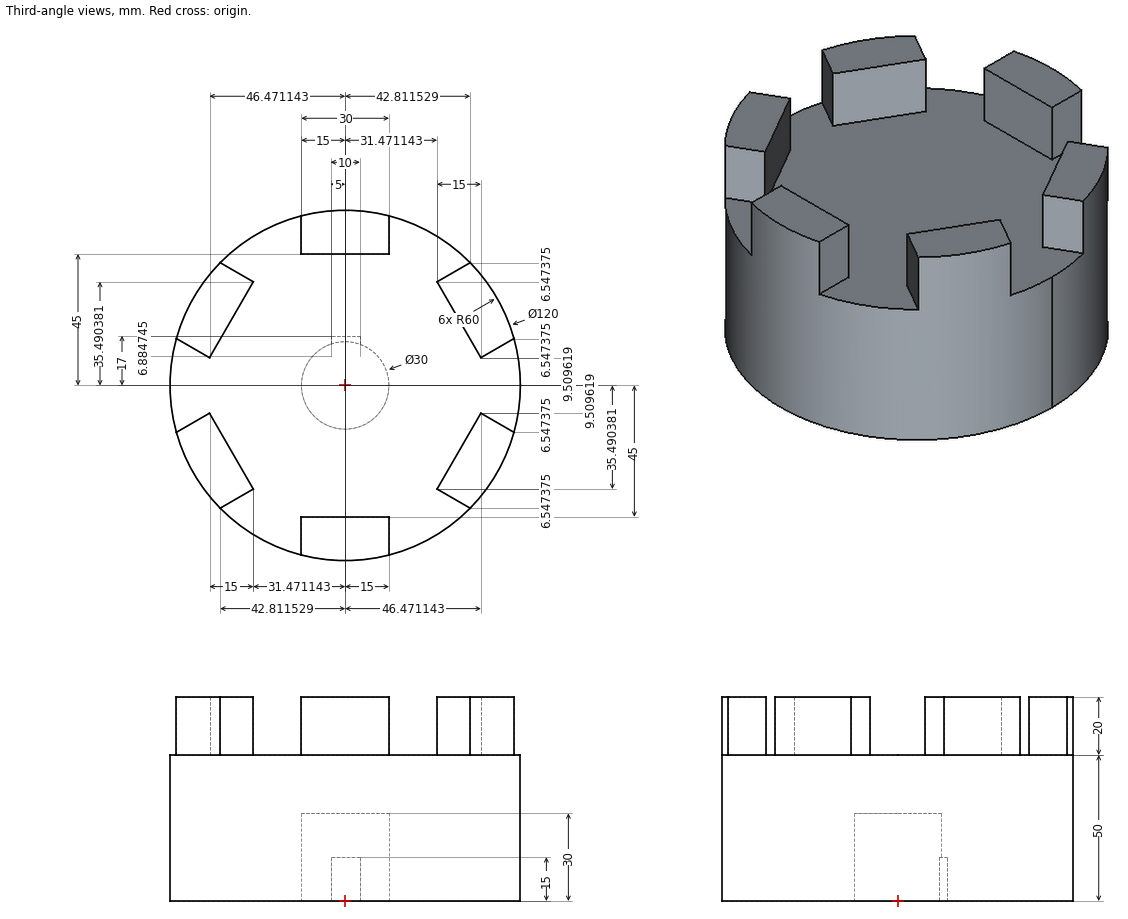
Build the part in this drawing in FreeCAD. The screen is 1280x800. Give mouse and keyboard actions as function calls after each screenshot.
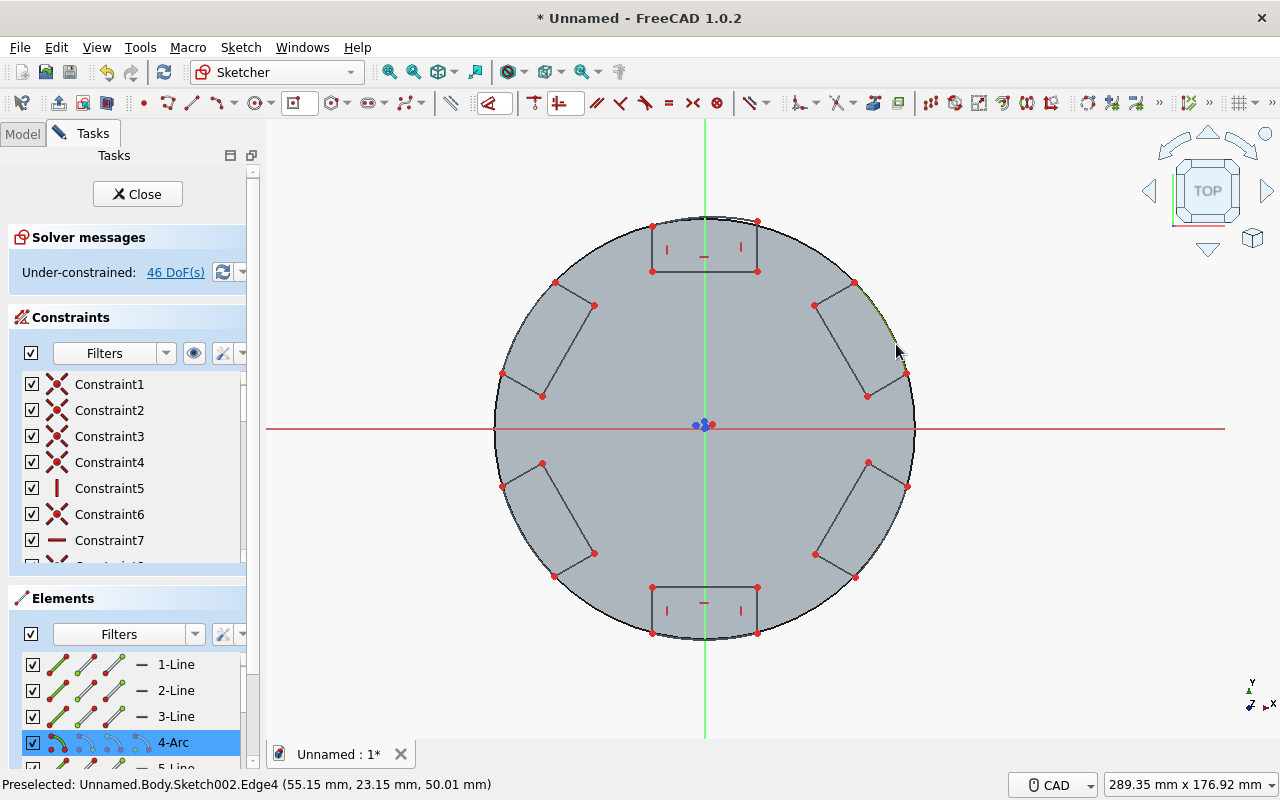
click(875, 552)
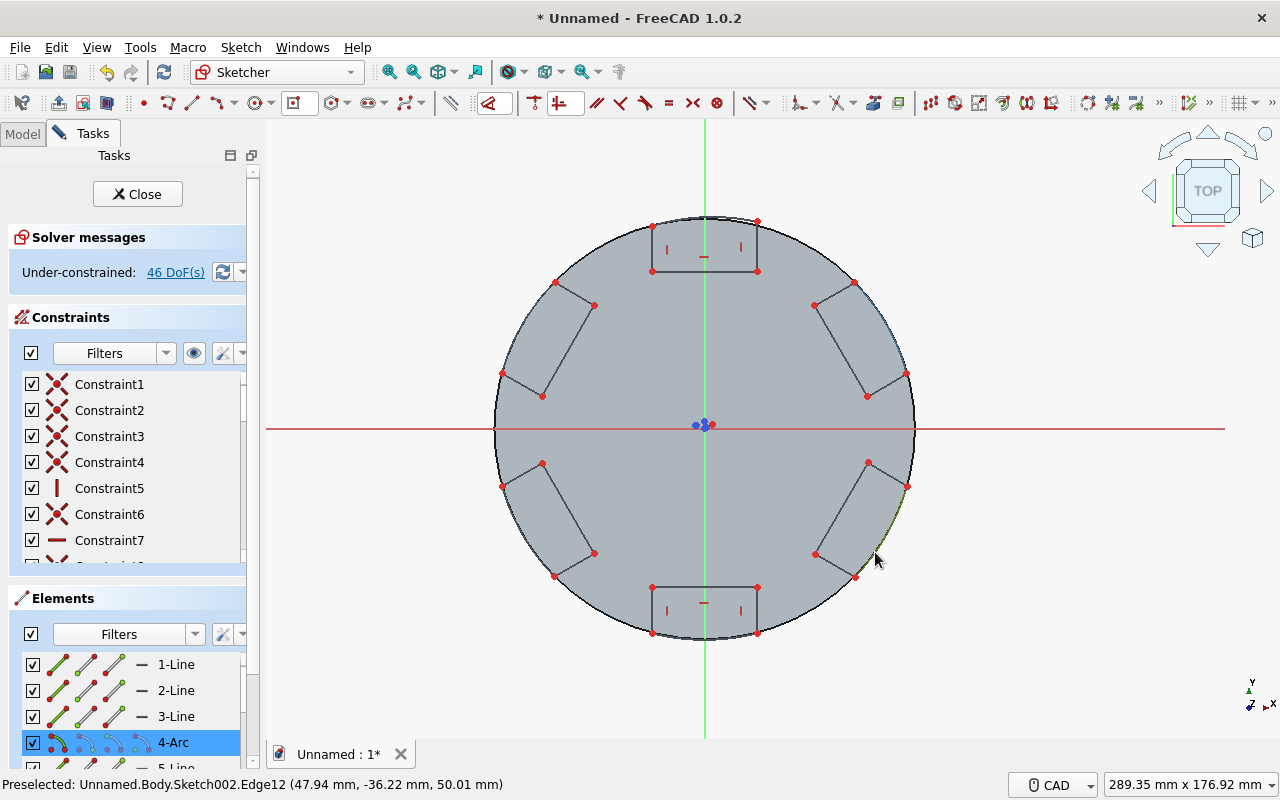
key(c)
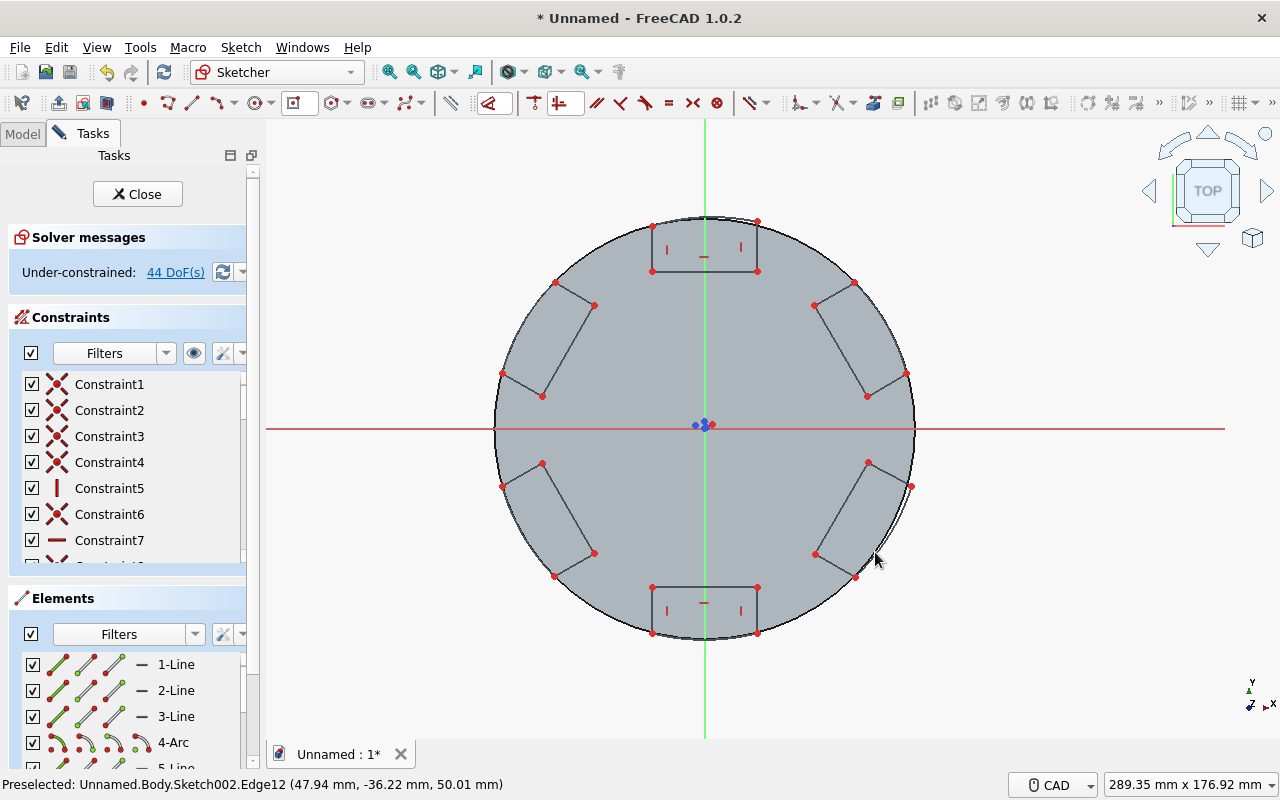
click(896, 344)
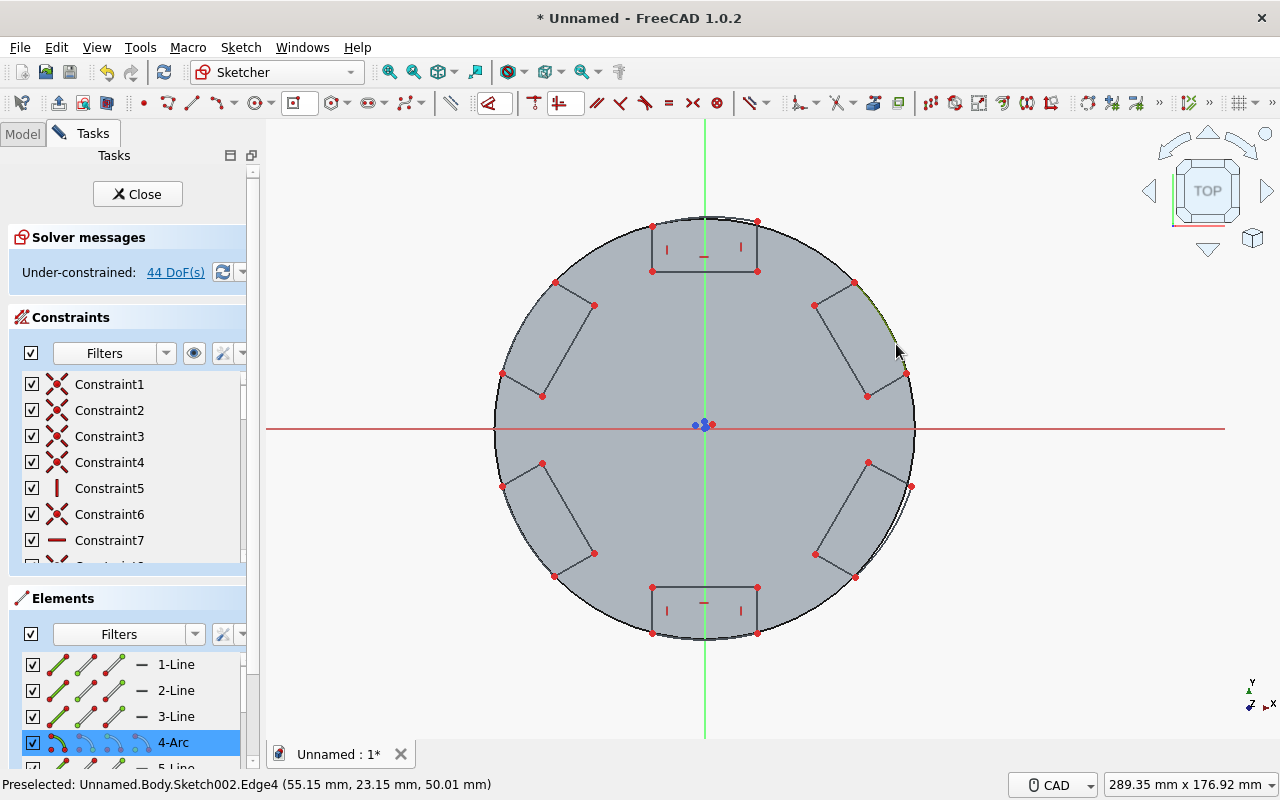
click(683, 639)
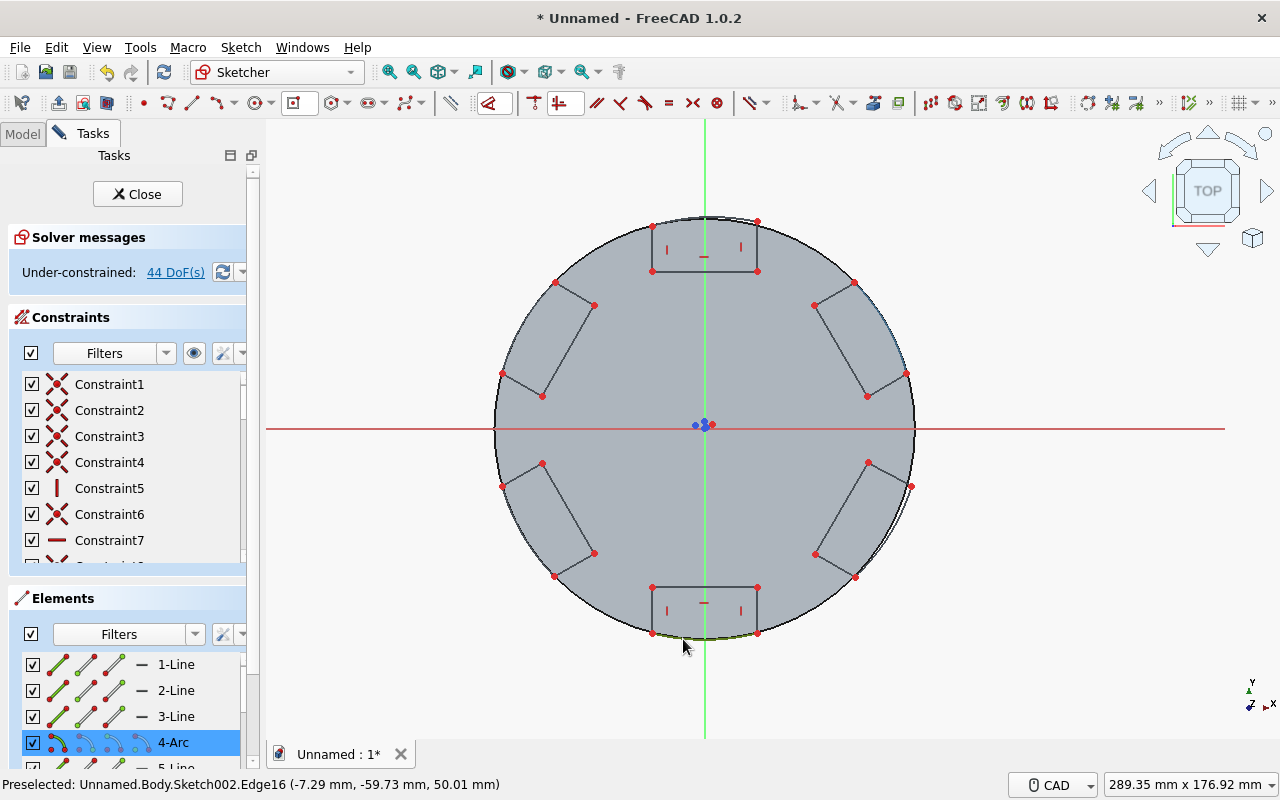
click(534, 104)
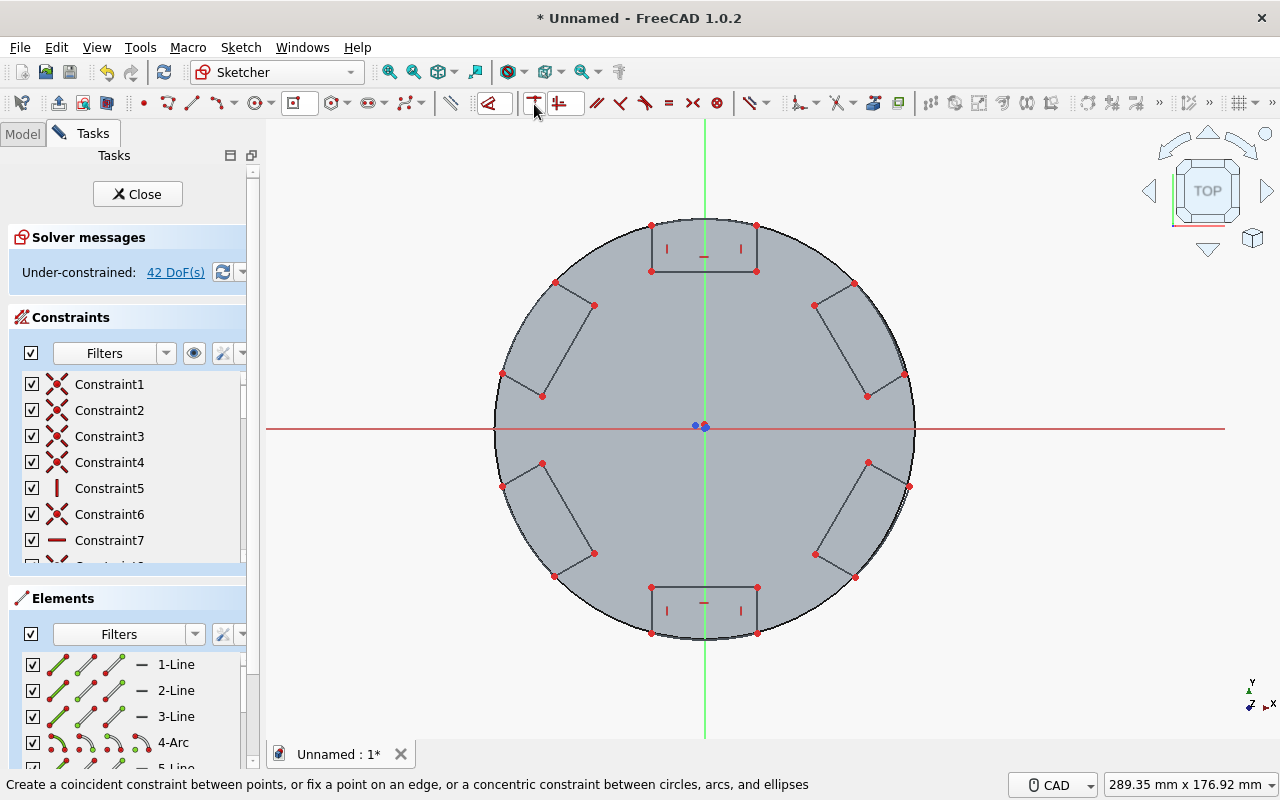
click(895, 344)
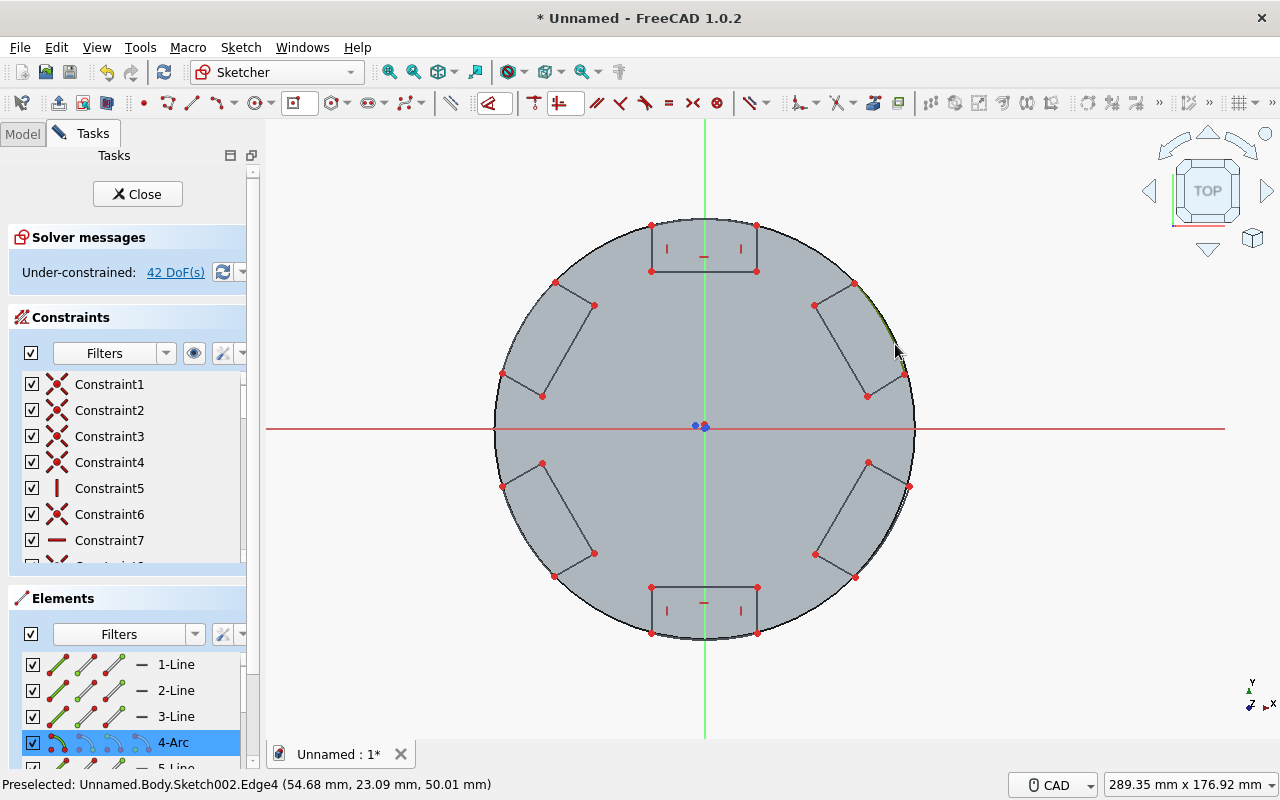
click(513, 516)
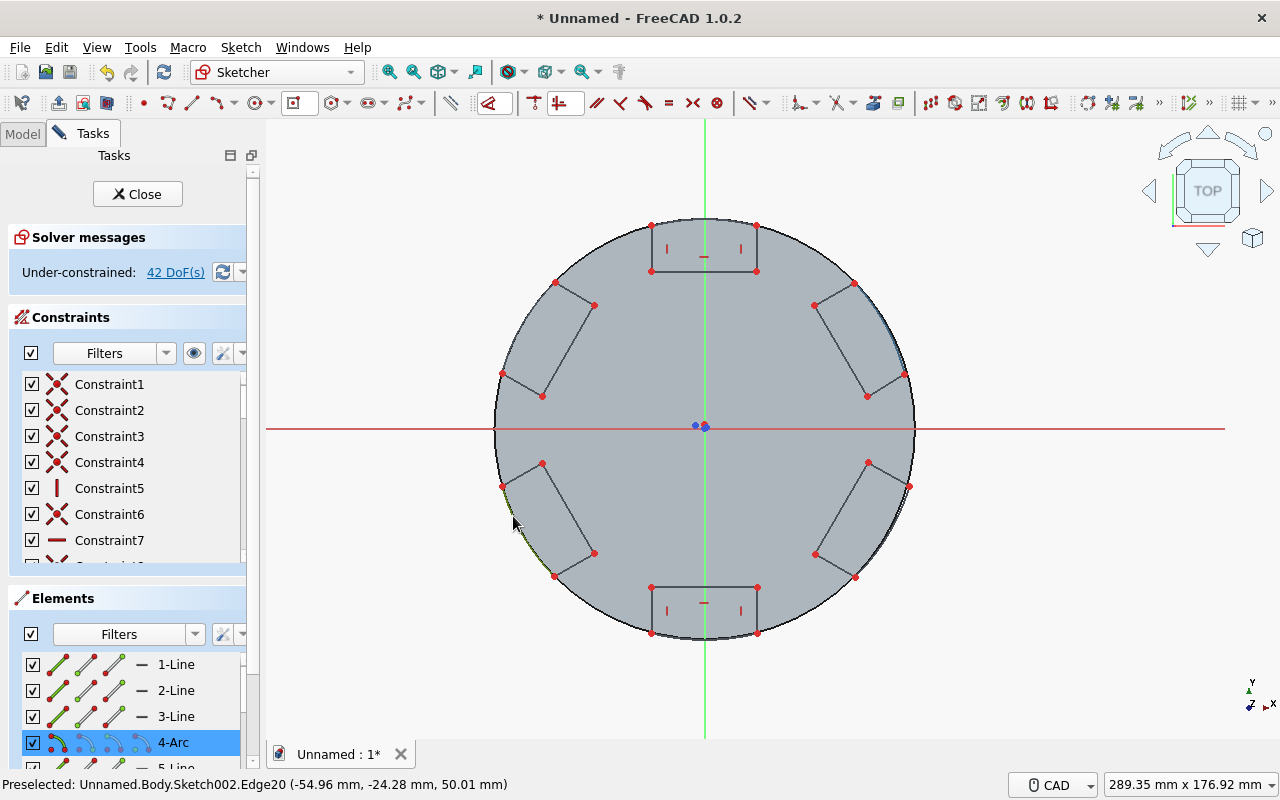
key(c)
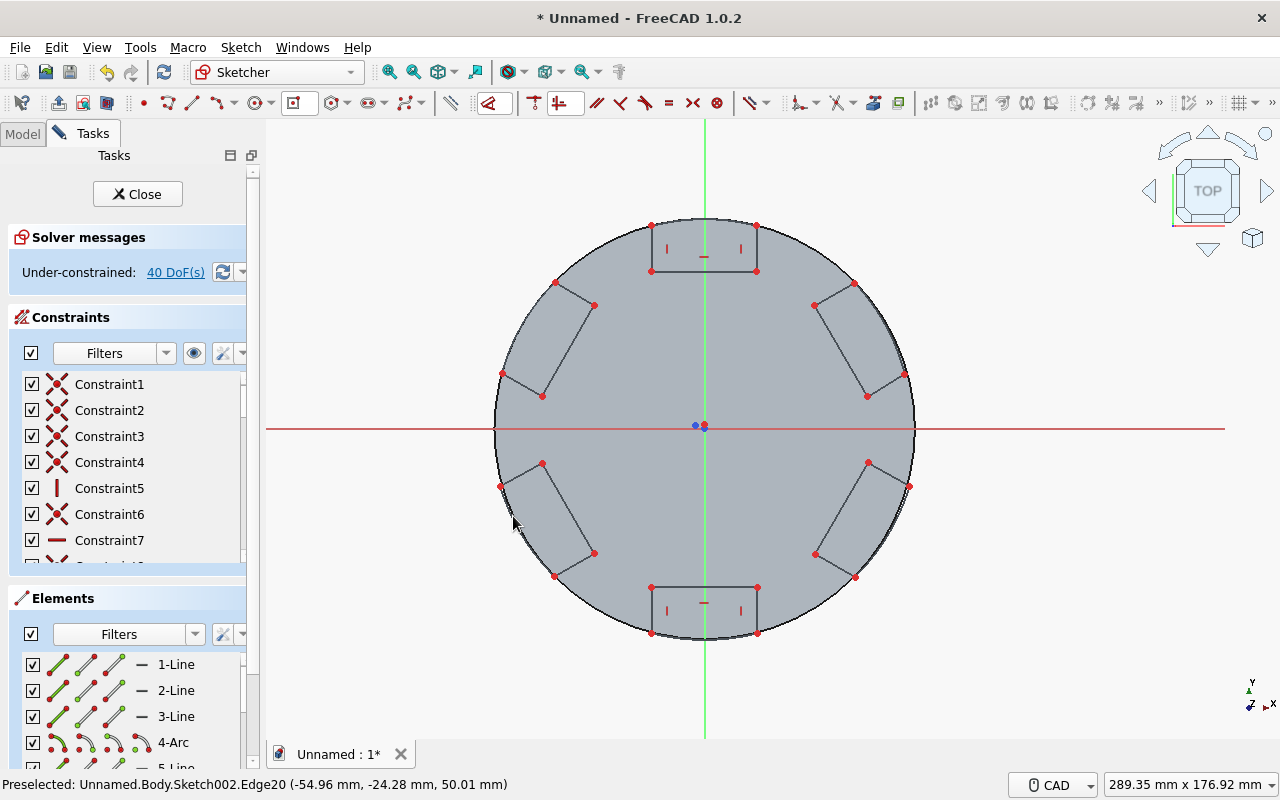
click(895, 344)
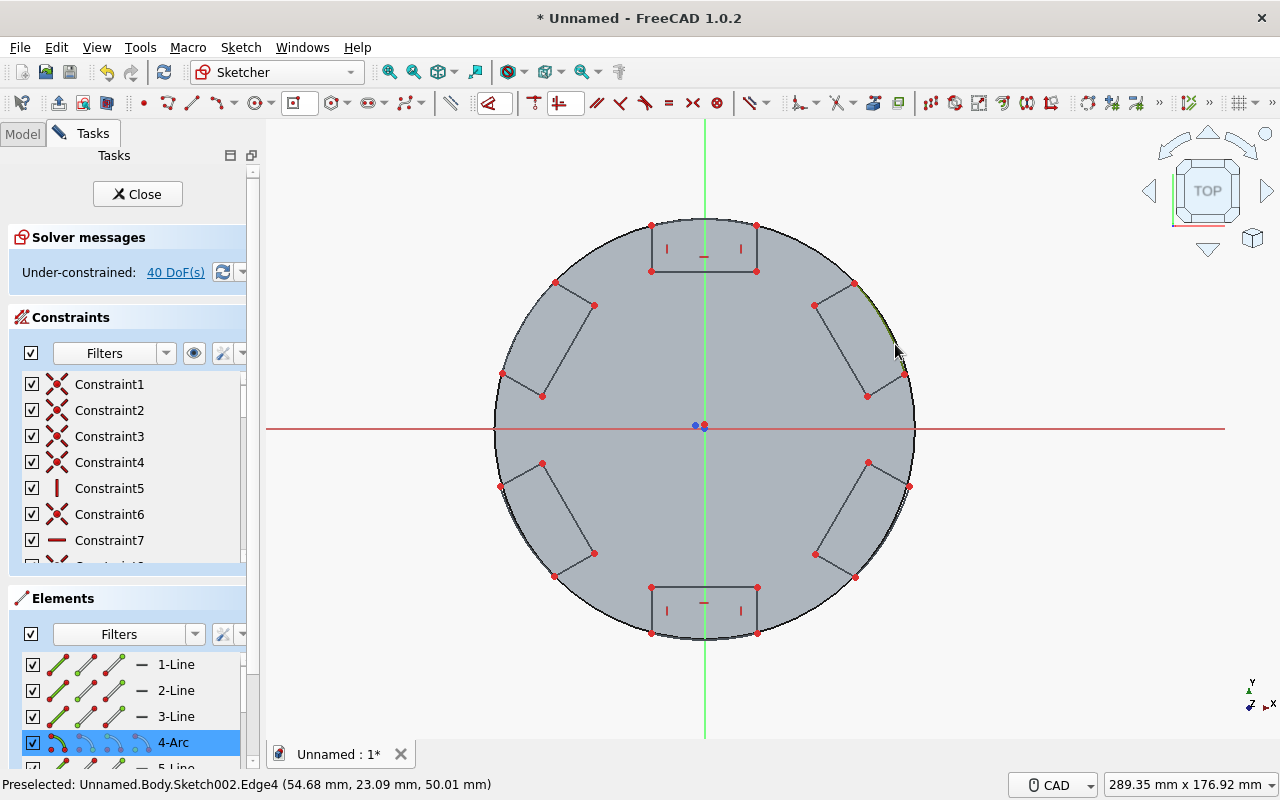
click(534, 307)